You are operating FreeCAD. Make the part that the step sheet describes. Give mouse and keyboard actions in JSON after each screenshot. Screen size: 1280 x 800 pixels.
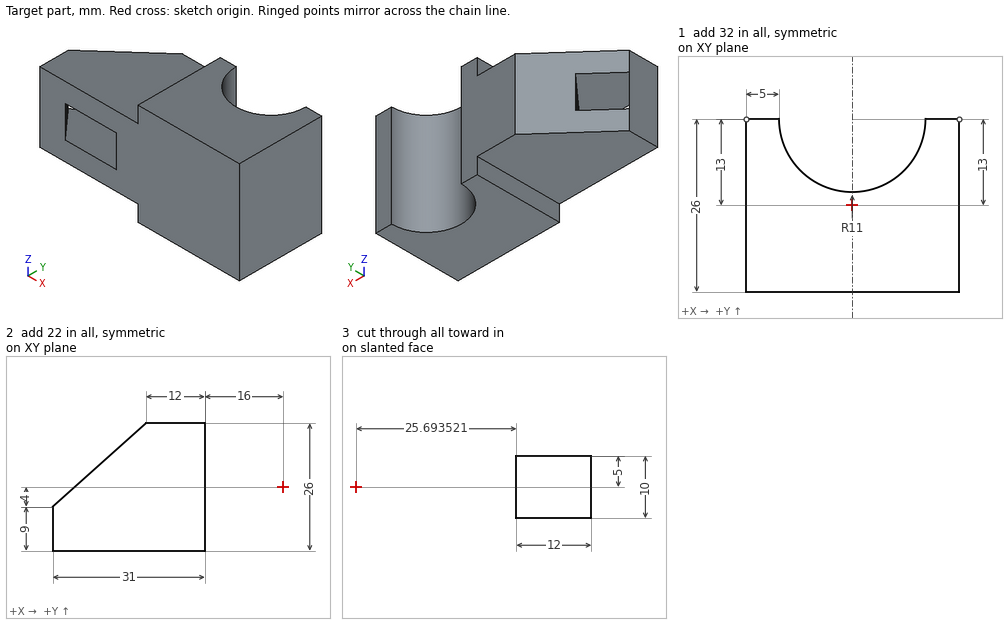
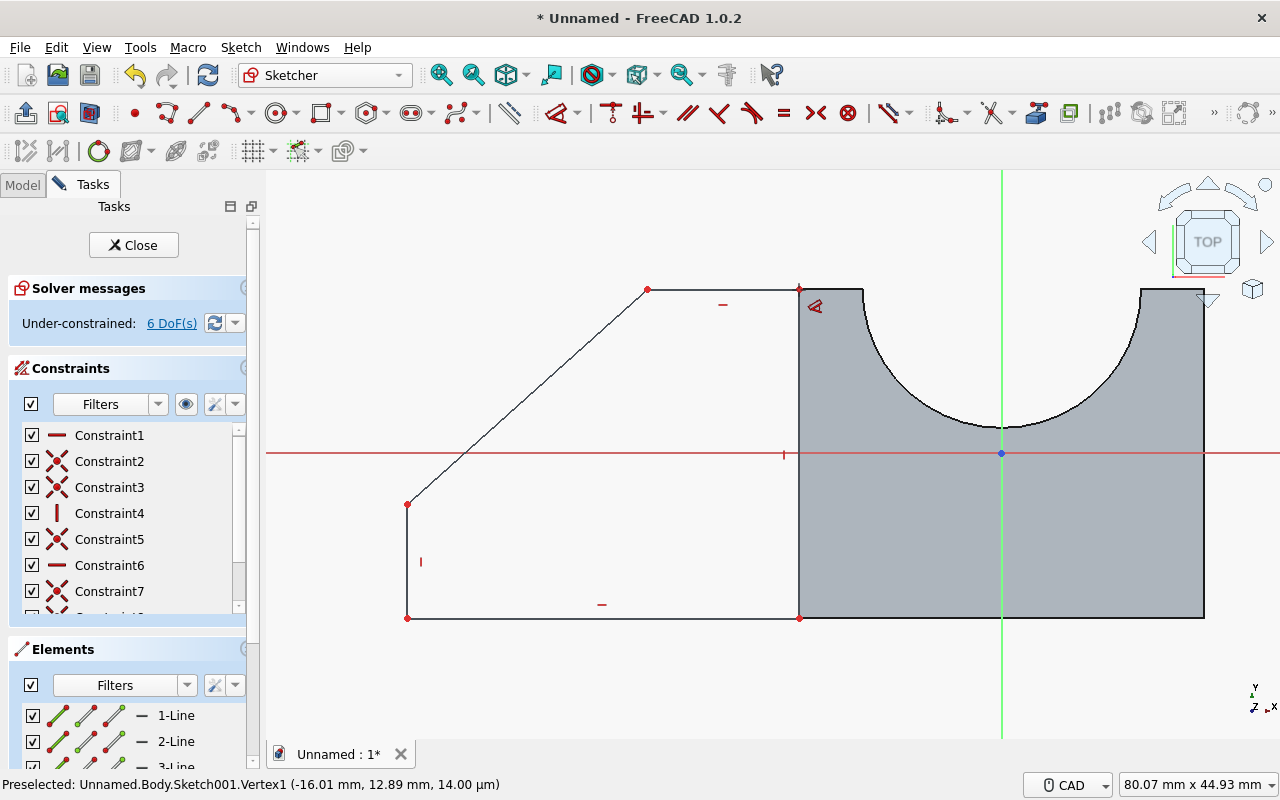
{"action": "left_click", "coordinate": [407, 539]}
{"action": "left_click", "coordinate": [373, 562]}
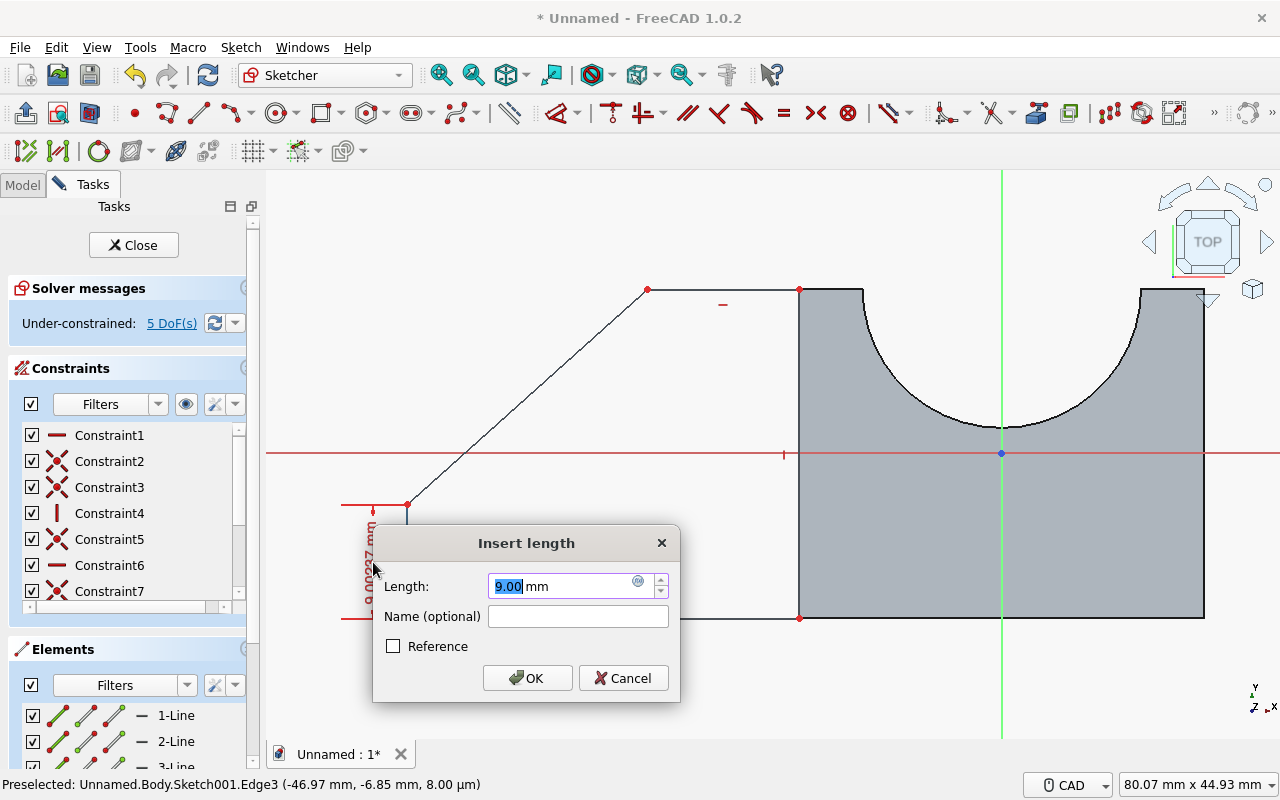
{"action": "type", "text": "9"}
{"action": "key", "text": "Return"}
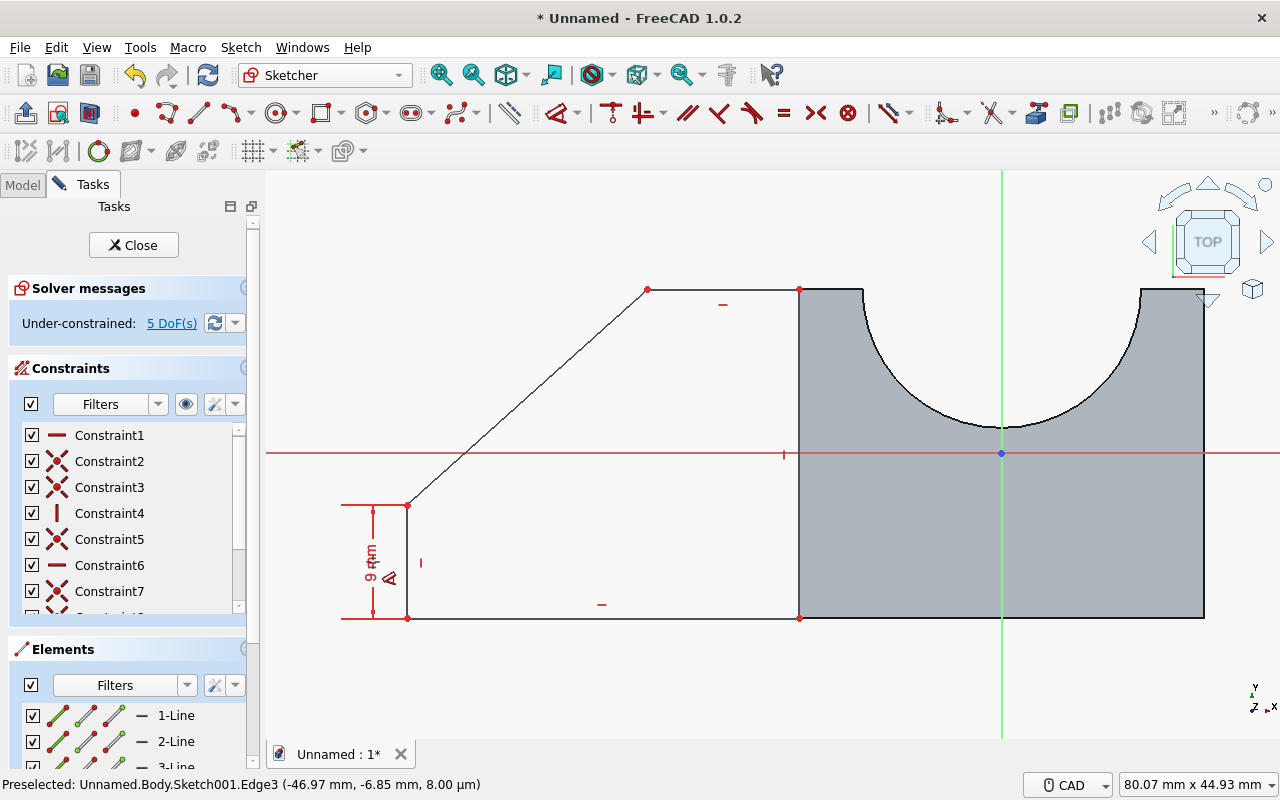
{"action": "left_click", "coordinate": [753, 290]}
{"action": "left_click", "coordinate": [723, 256]}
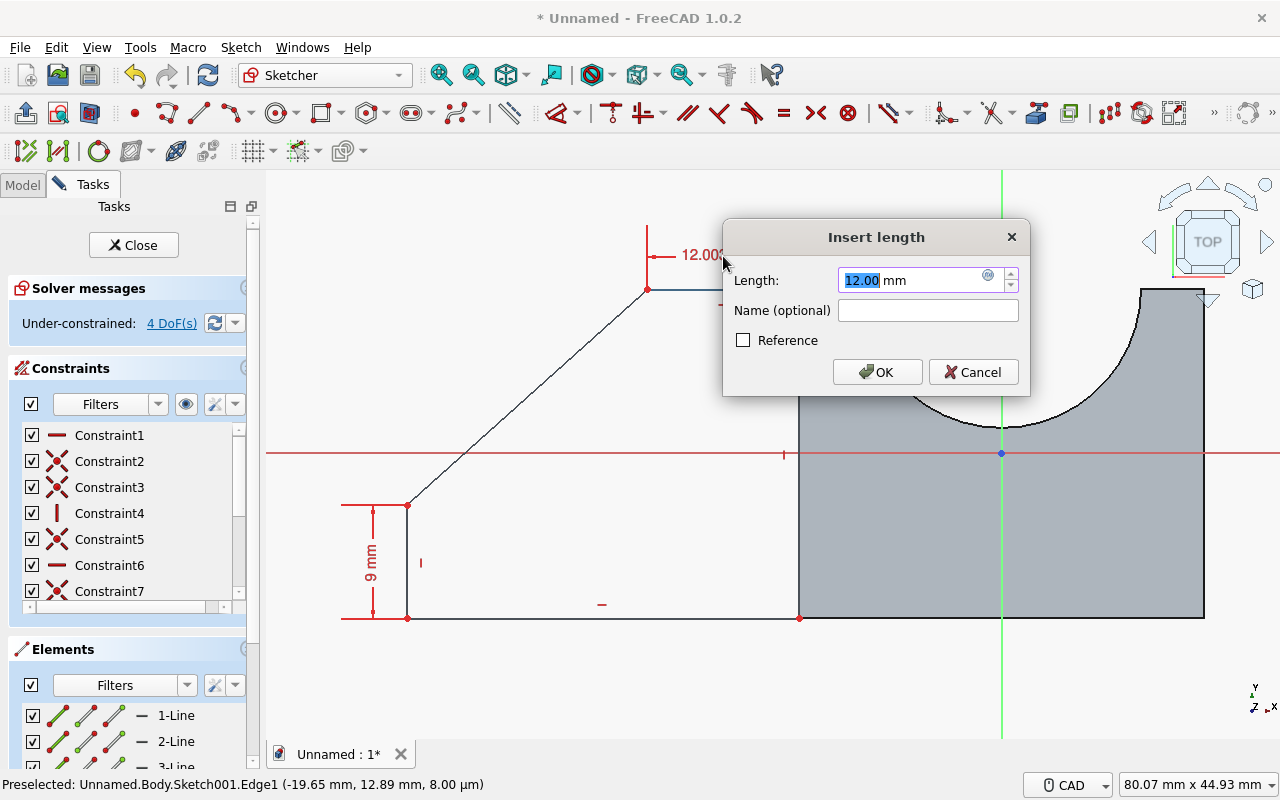
{"action": "type", "text": "12"}
{"action": "key", "text": "Return"}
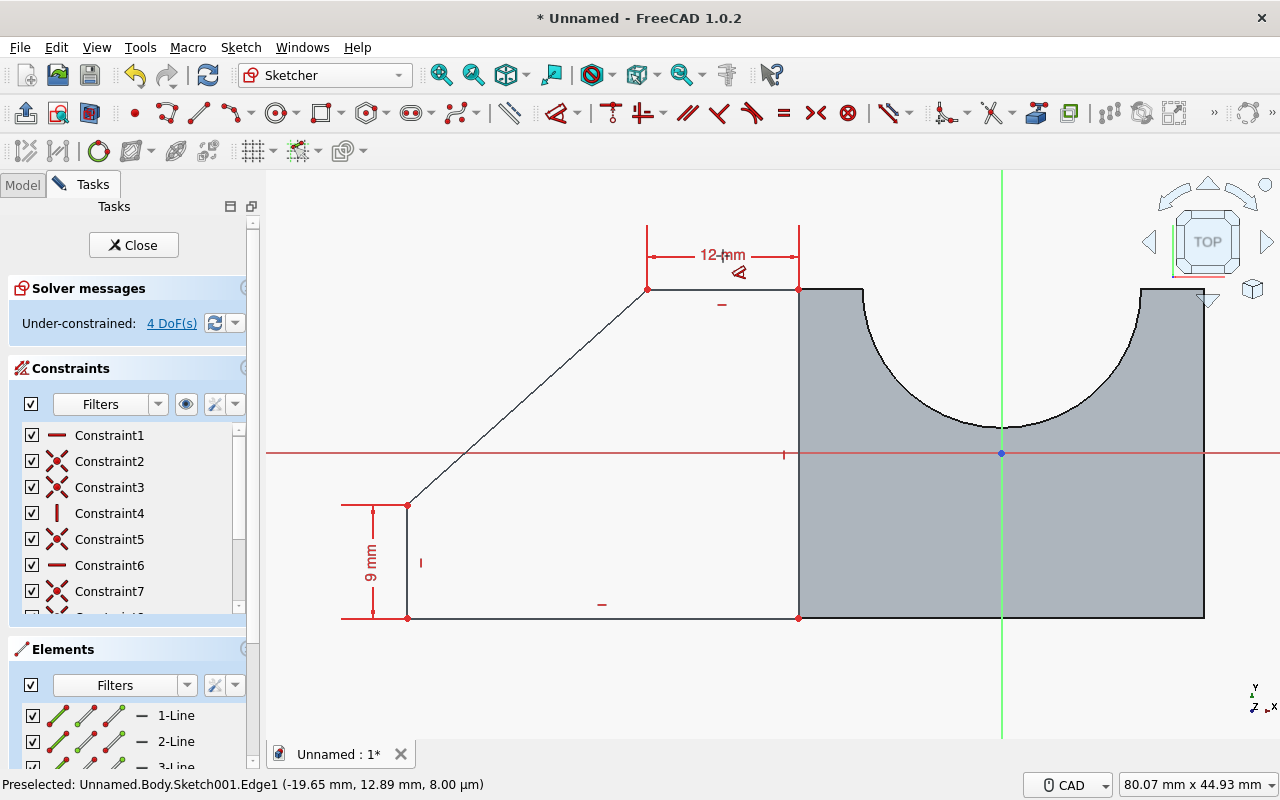
{"action": "left_click", "coordinate": [525, 619]}
{"action": "left_click", "coordinate": [603, 653]}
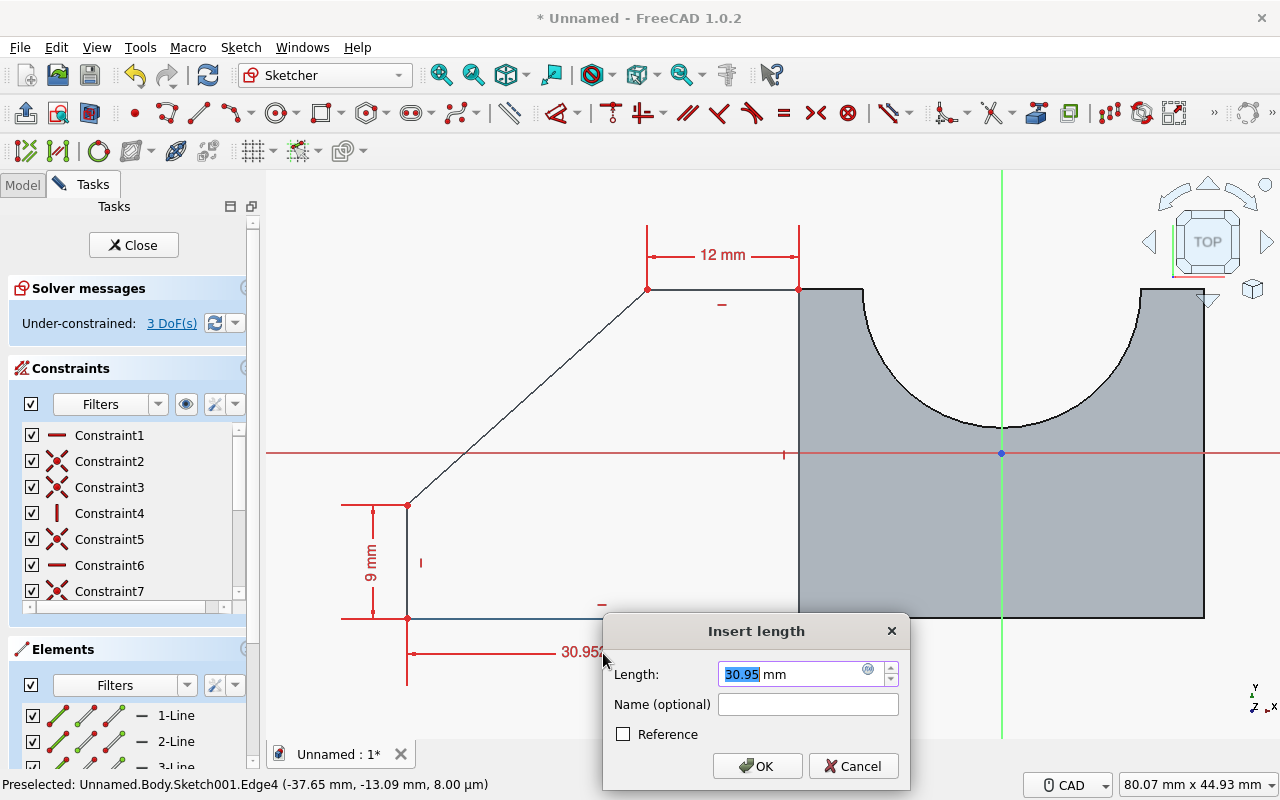
{"action": "type", "text": "31"}
{"action": "key", "text": "Return"}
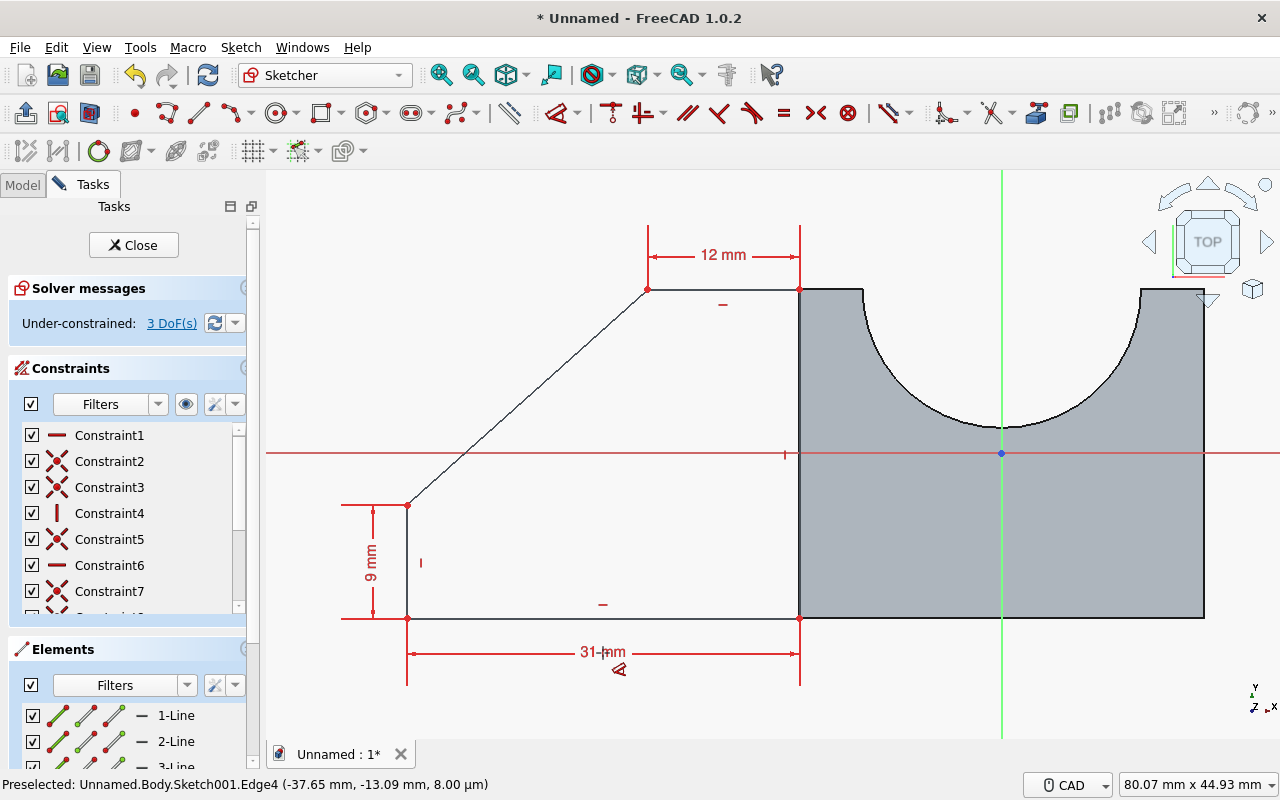
{"action": "left_click", "coordinate": [800, 520]}
{"action": "left_click", "coordinate": [834, 379]}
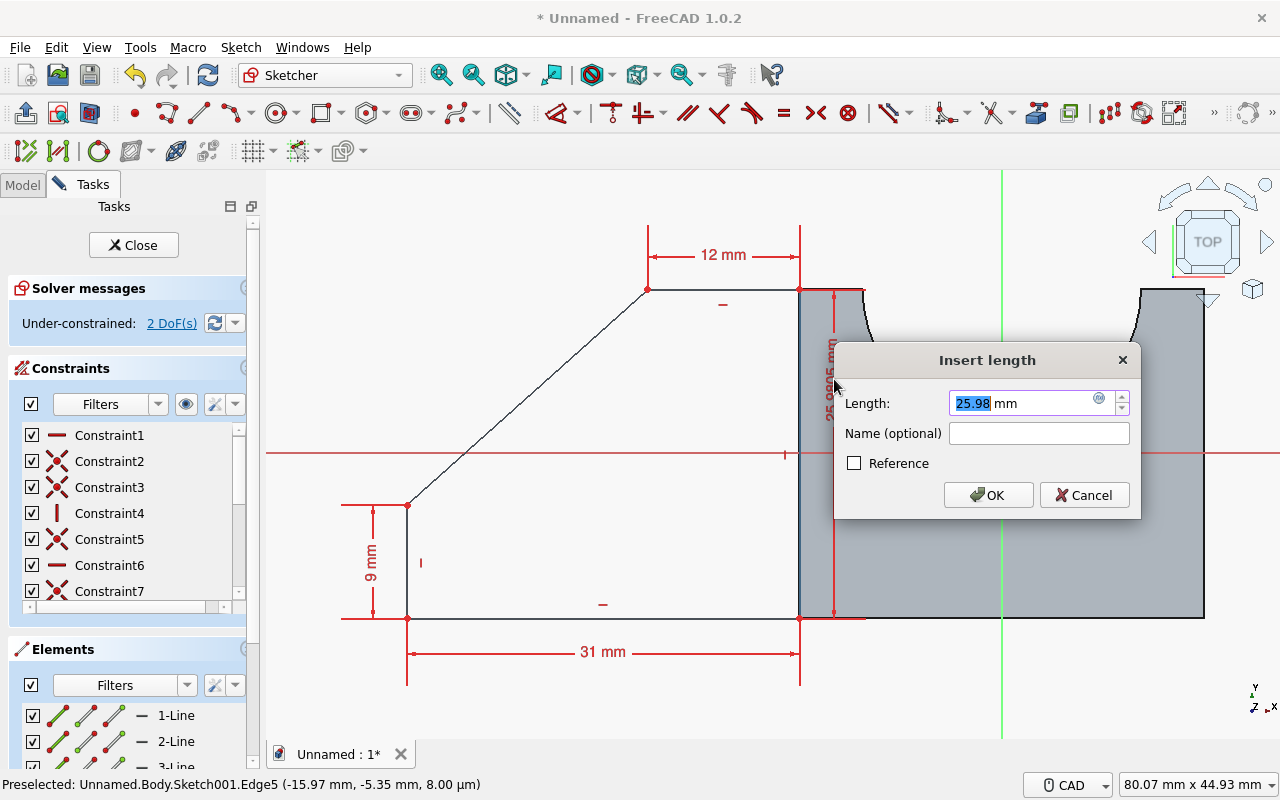
{"action": "type", "text": "26"}
{"action": "key", "text": "Return"}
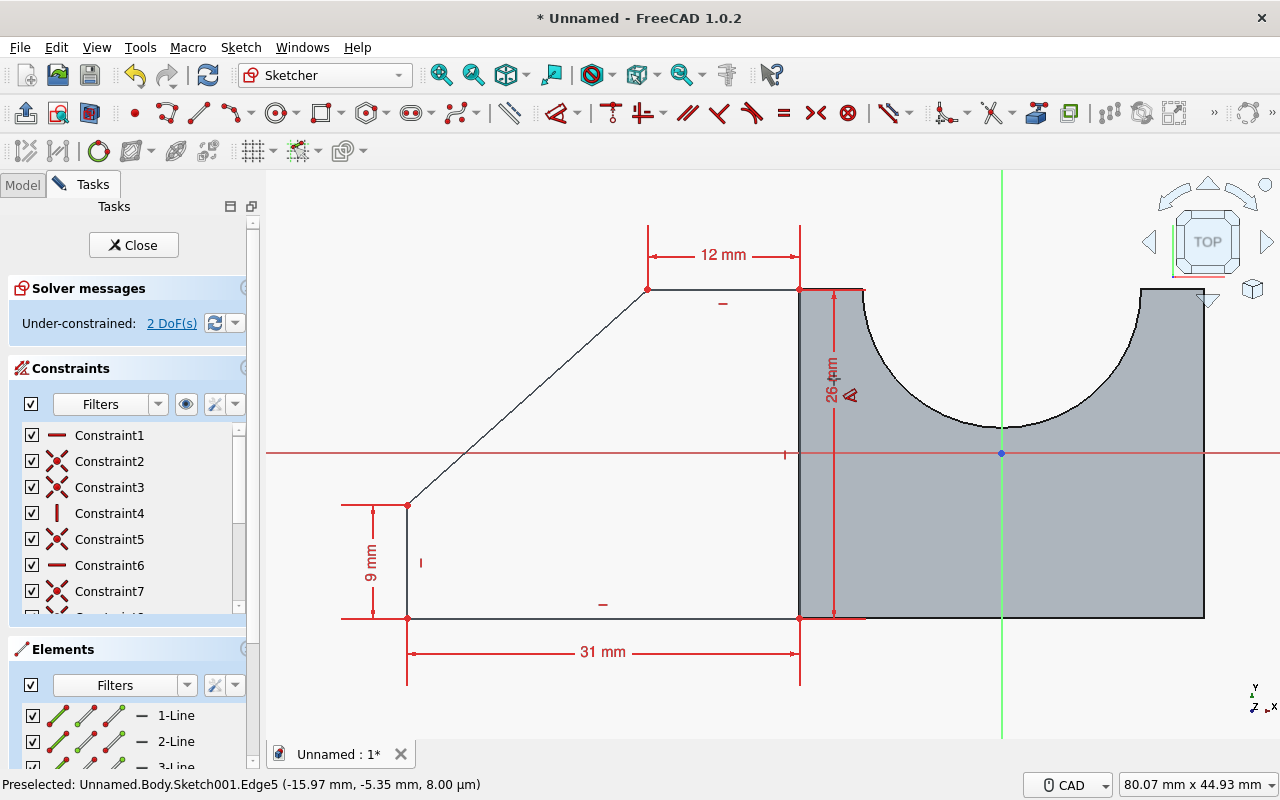
{"action": "left_click", "coordinate": [407, 505]}
{"action": "left_click", "coordinate": [1036, 479]}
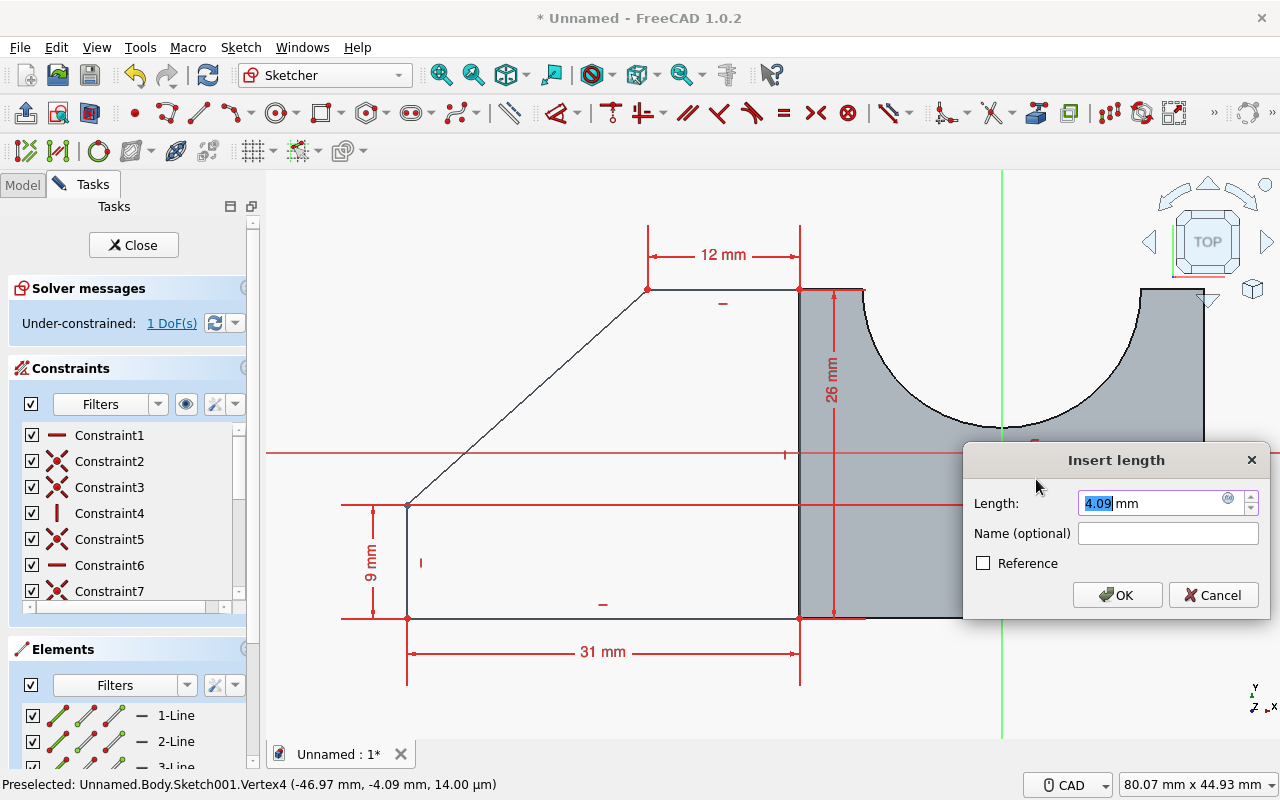
{"action": "type", "text": "4"}
{"action": "key", "text": "Return"}